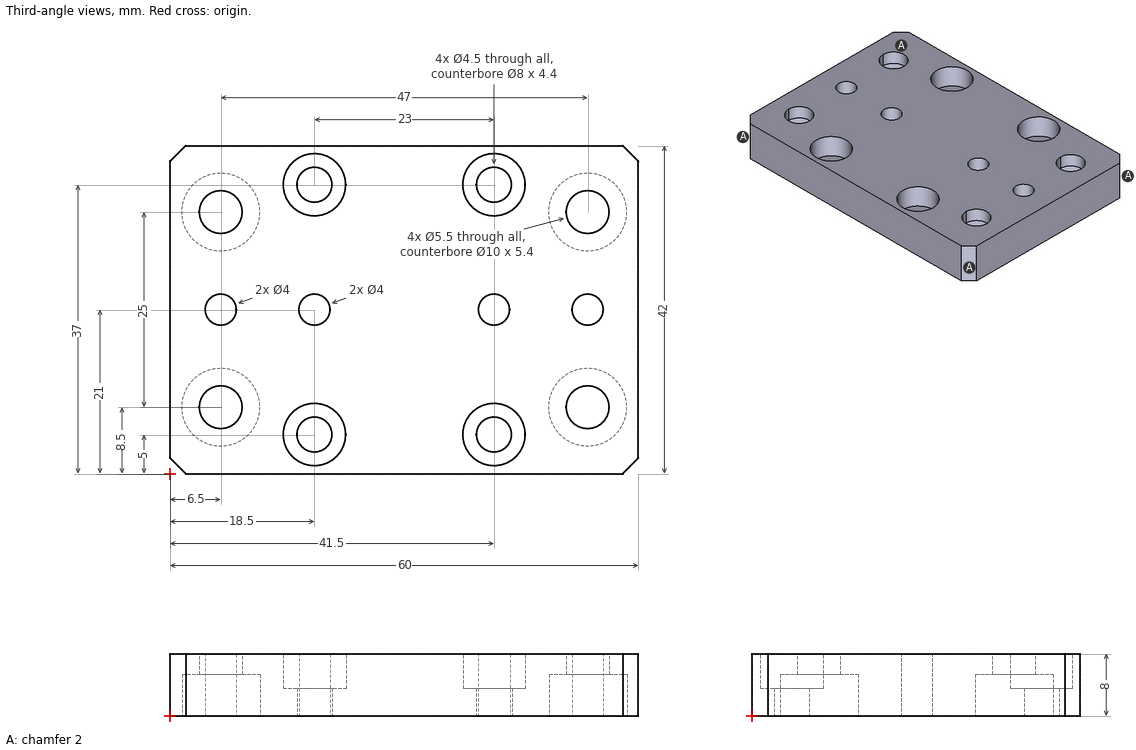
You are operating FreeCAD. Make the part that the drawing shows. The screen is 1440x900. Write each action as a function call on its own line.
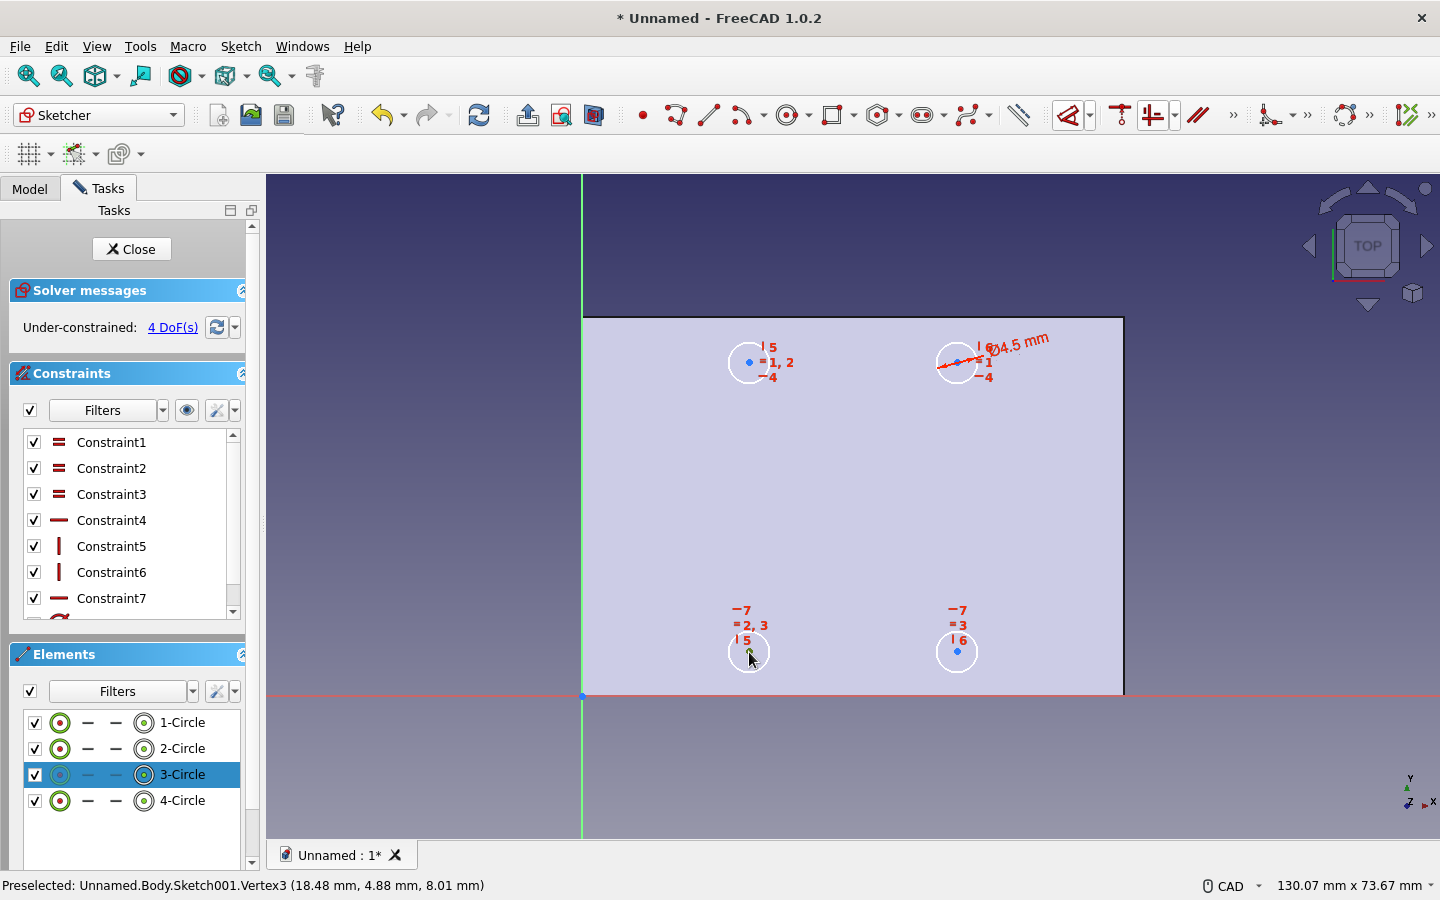
click(1090, 116)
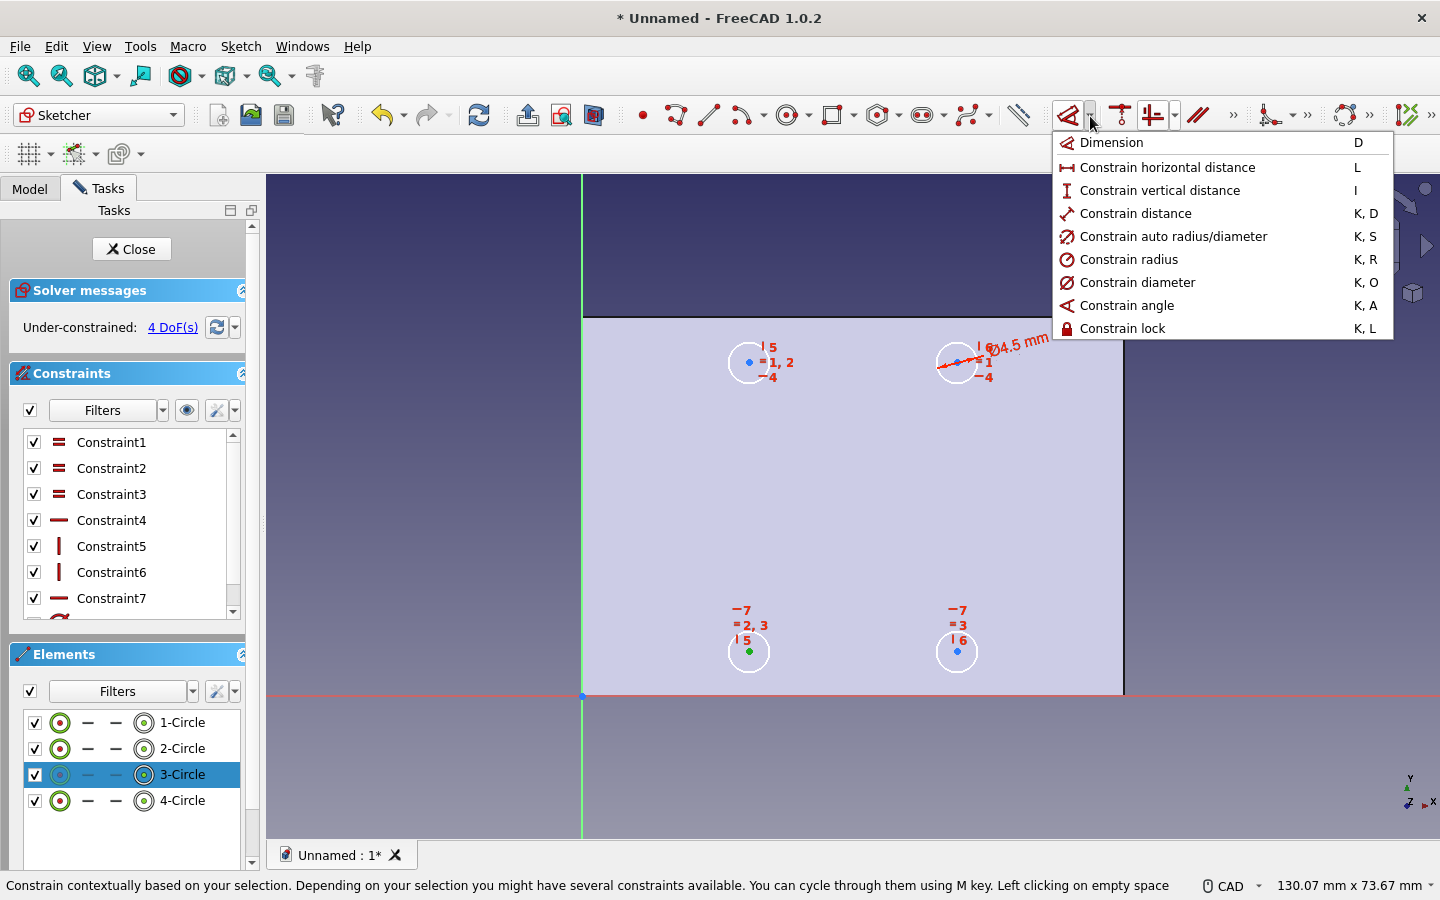
click(1223, 190)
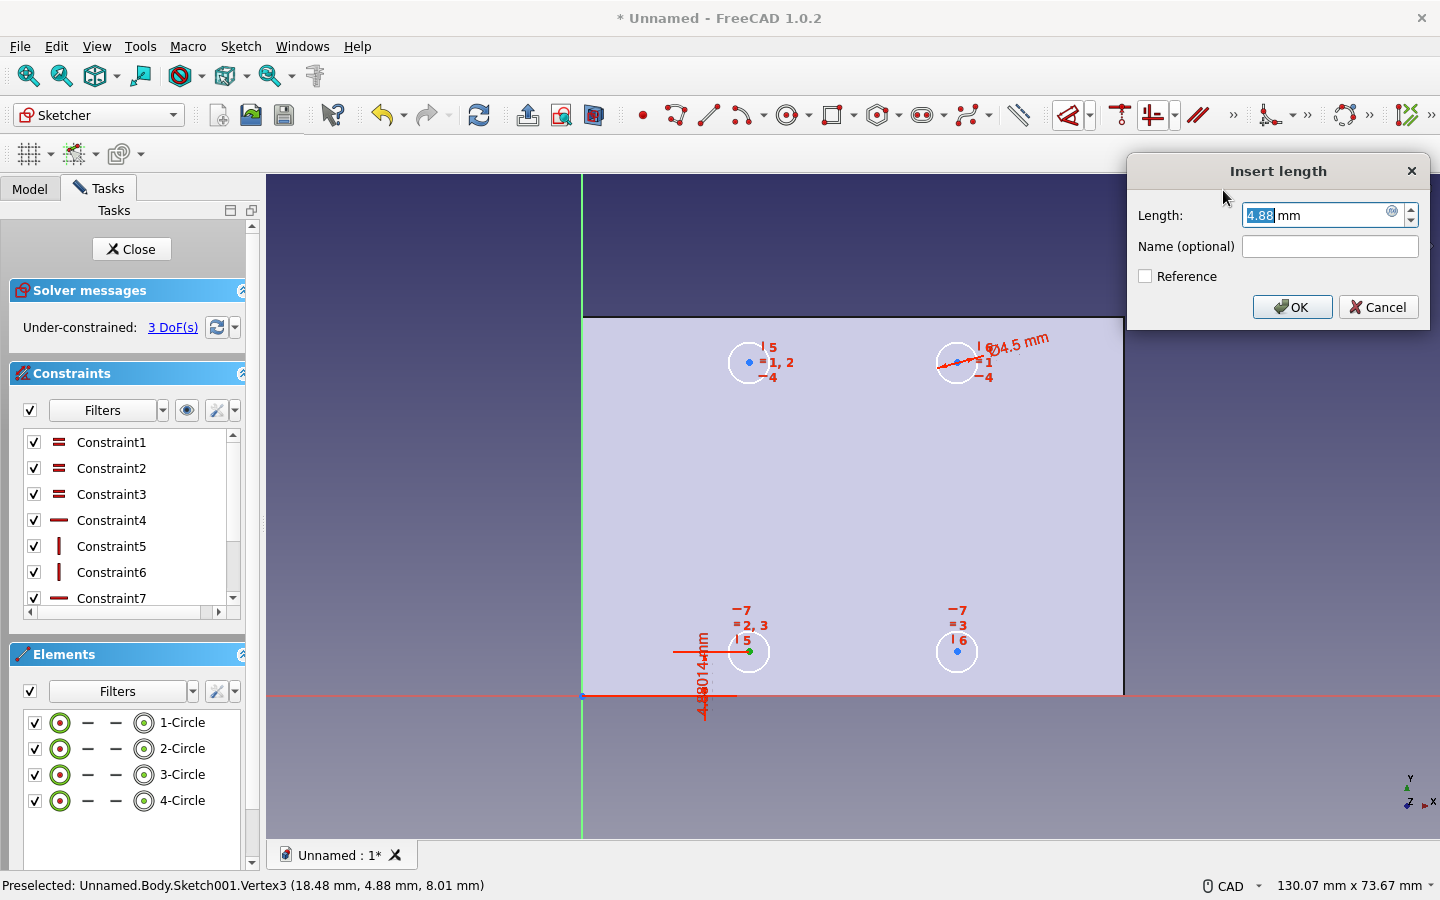
text(5)
key(Return)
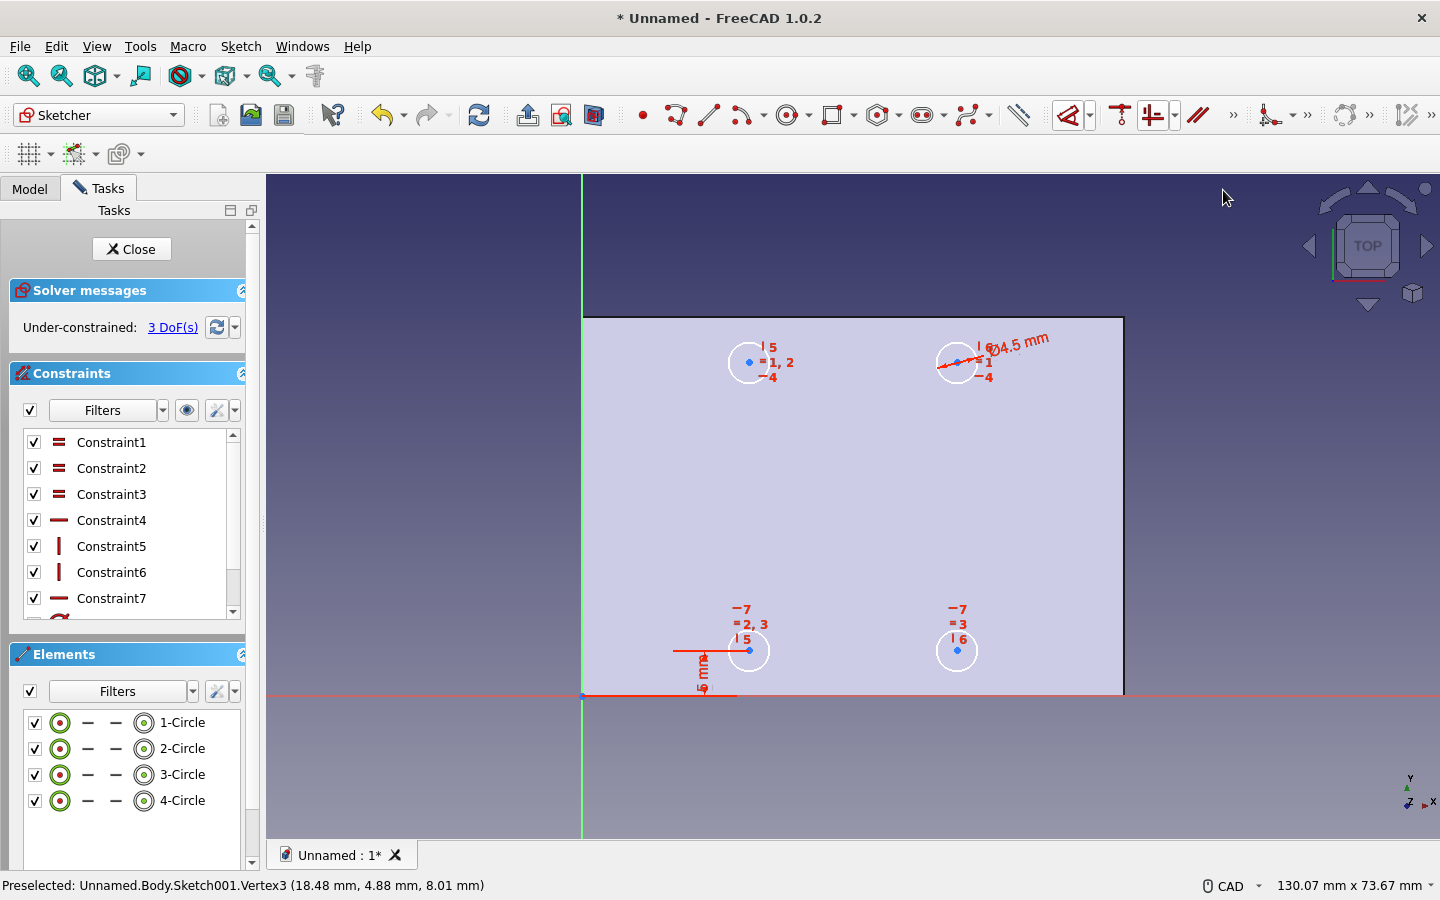
click(957, 363)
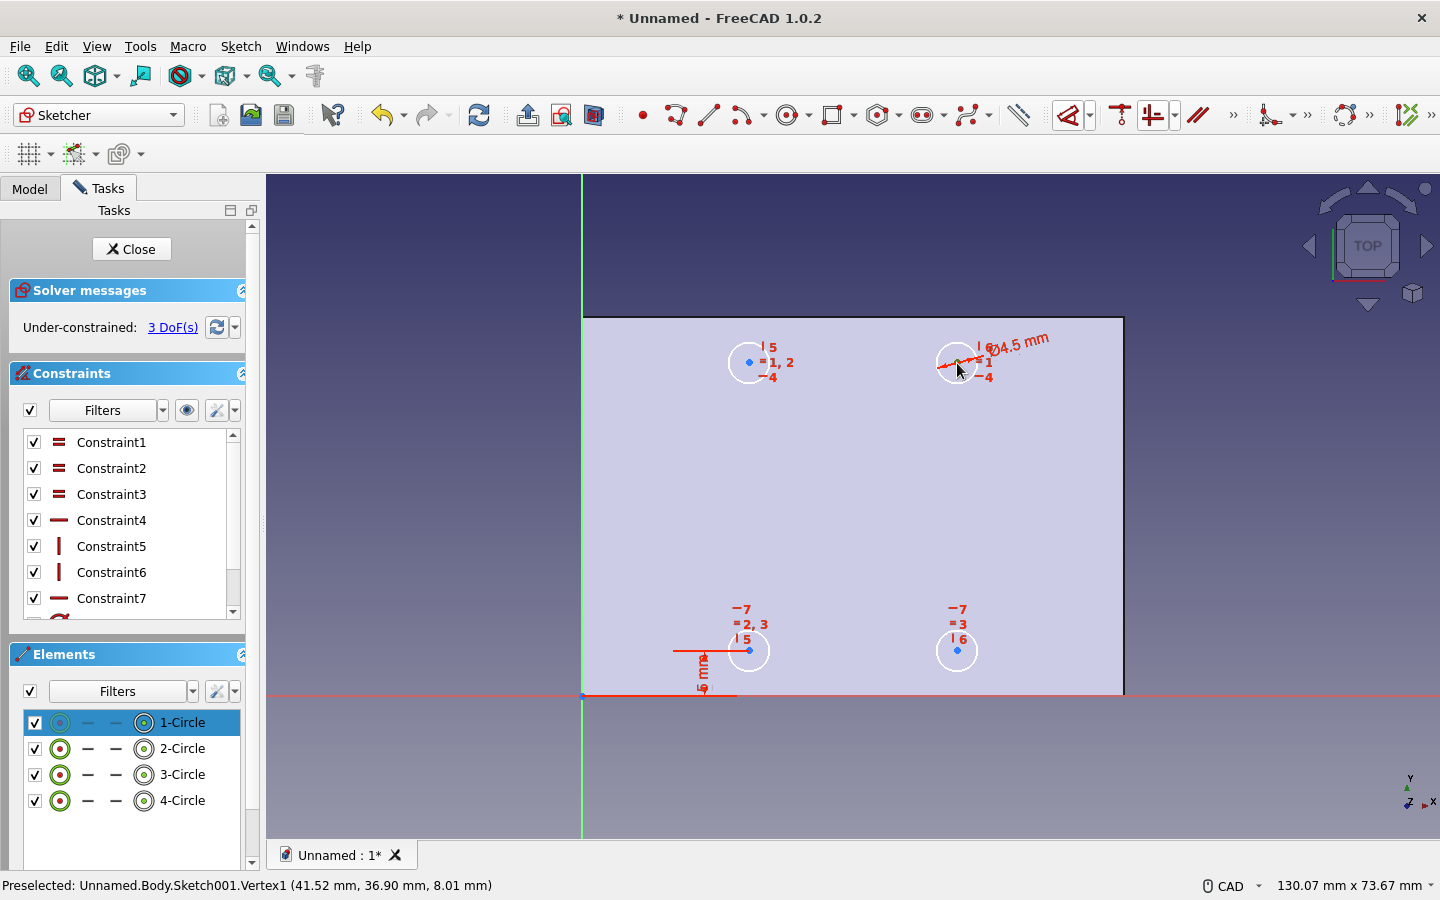
click(1090, 116)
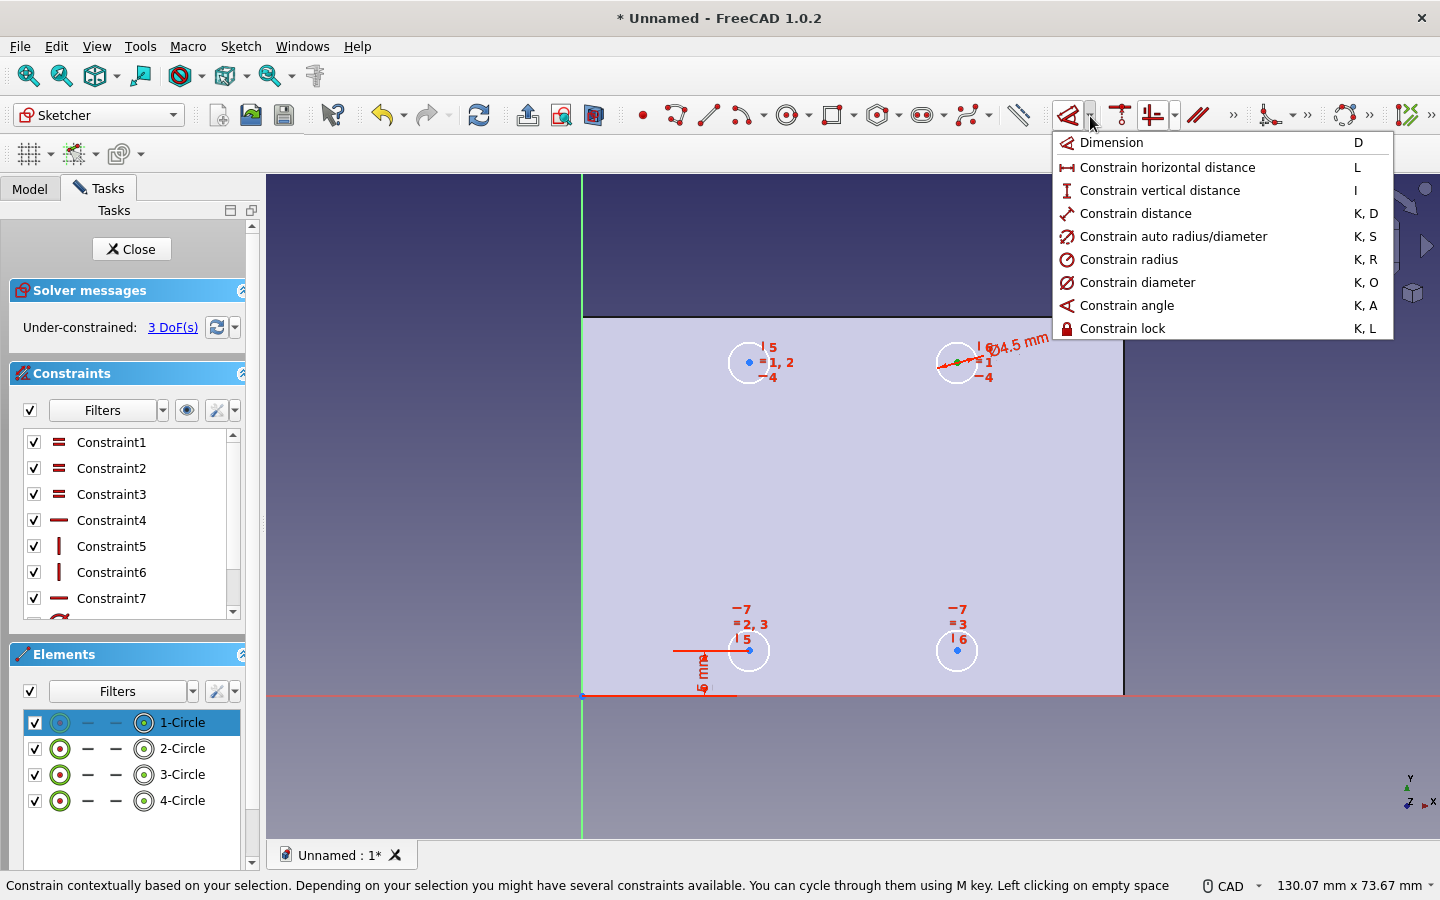
click(1223, 190)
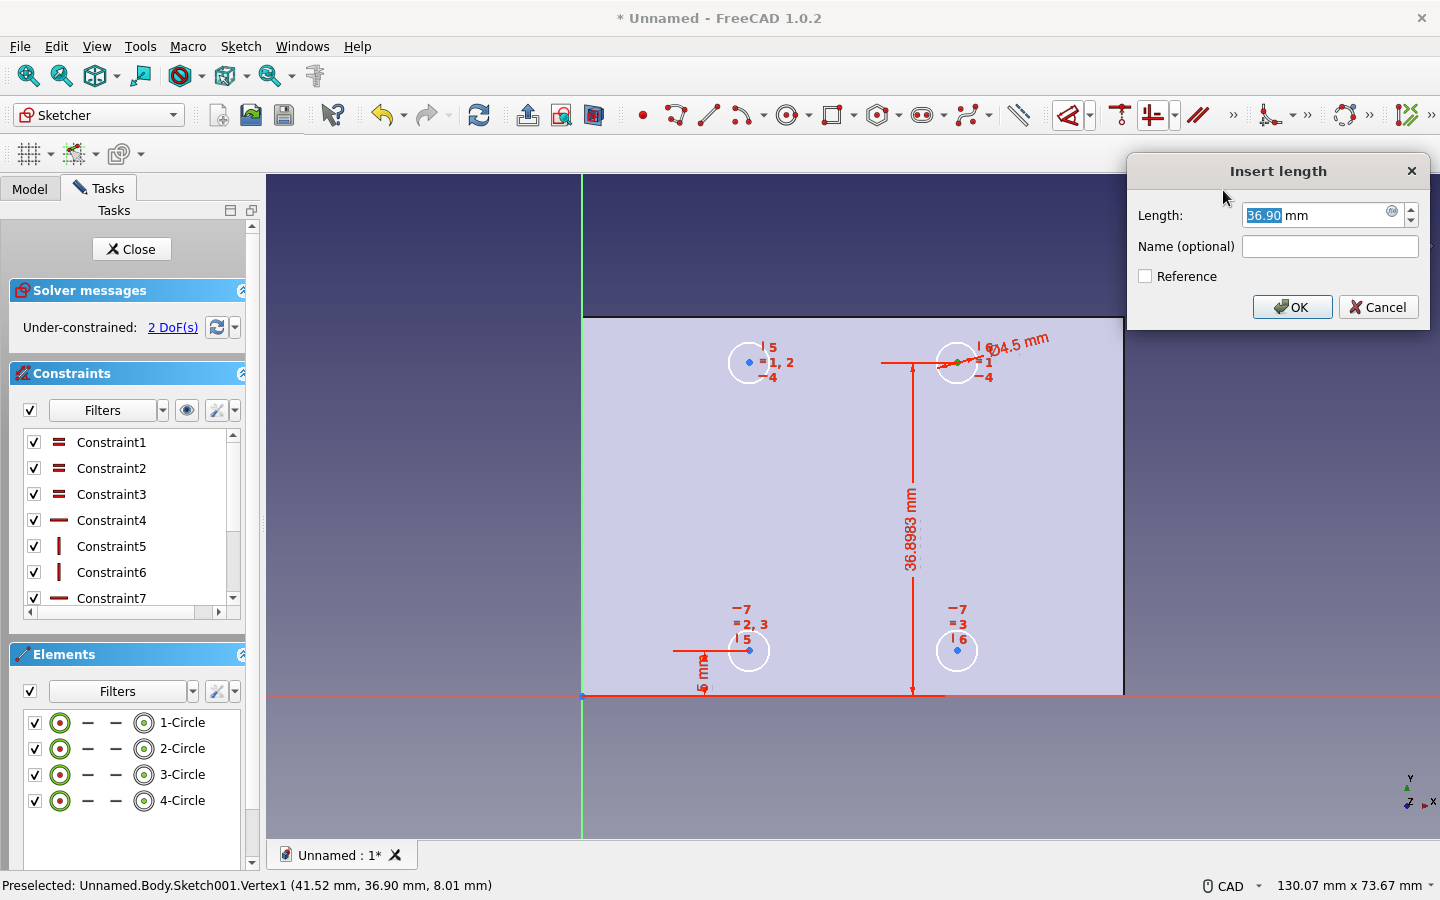
text(37)
key(Return)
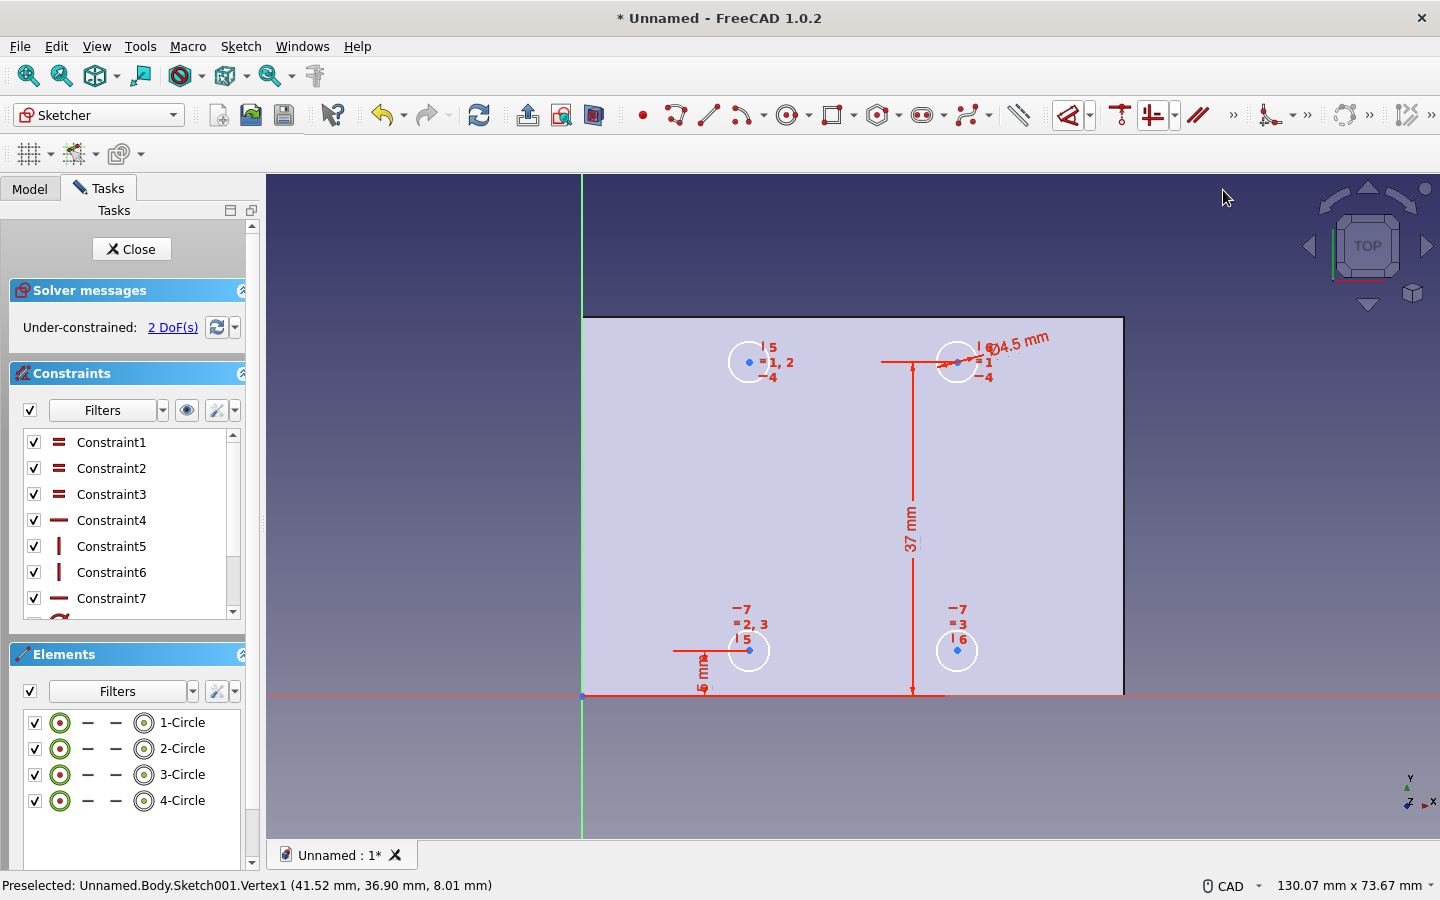
click(957, 362)